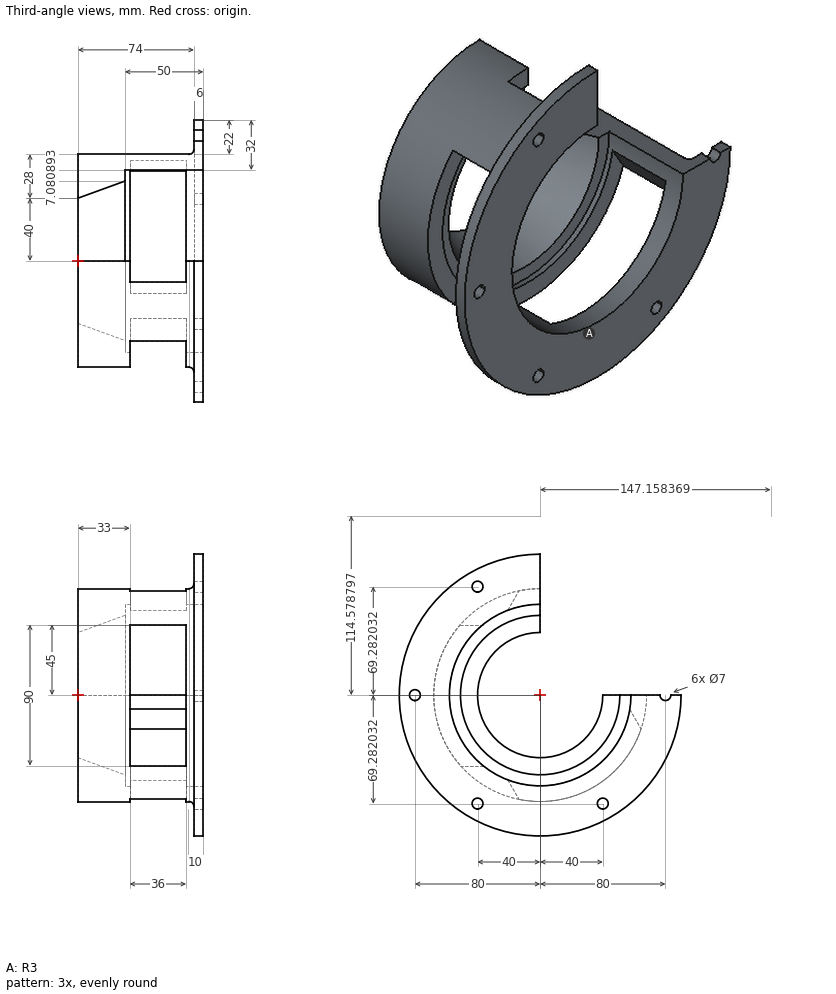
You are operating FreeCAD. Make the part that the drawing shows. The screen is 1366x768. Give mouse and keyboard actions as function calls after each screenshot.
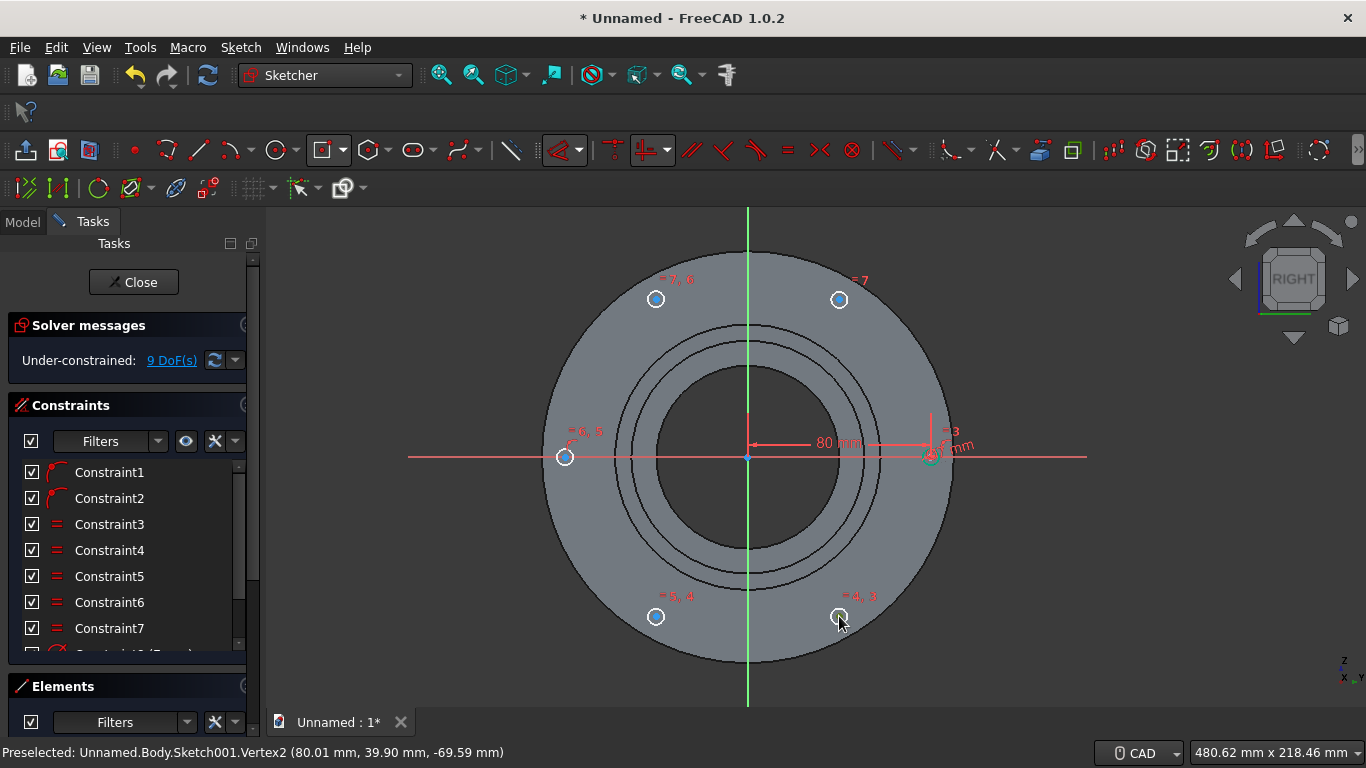
key(l)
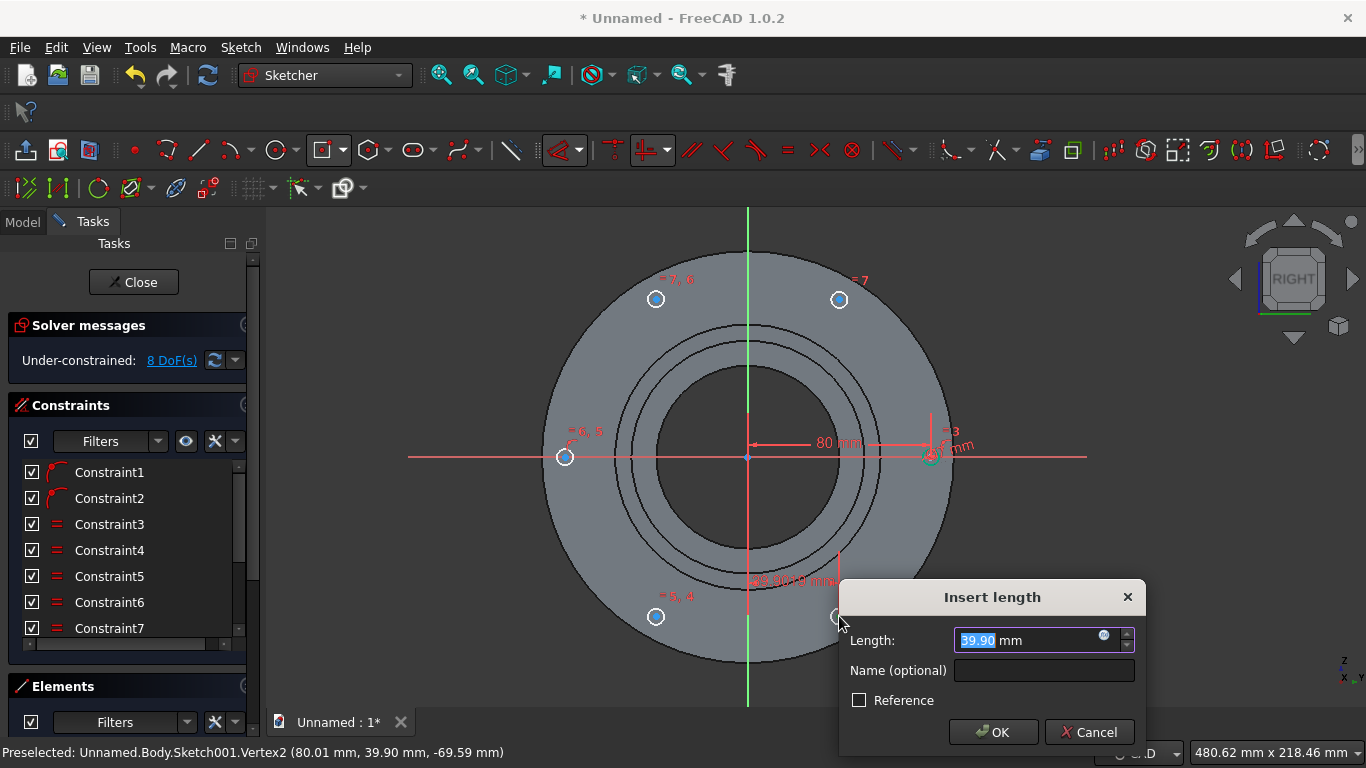
text(40)
key(Return)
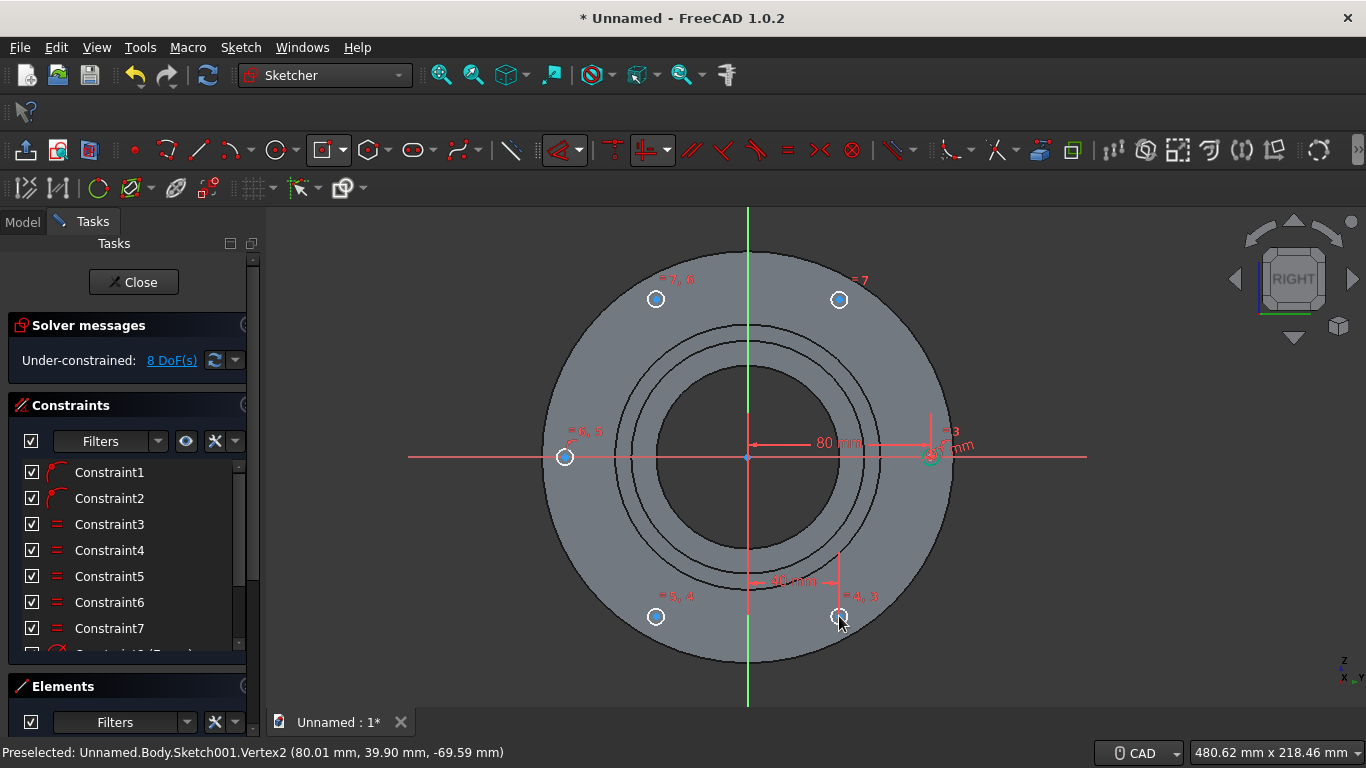
click(656, 617)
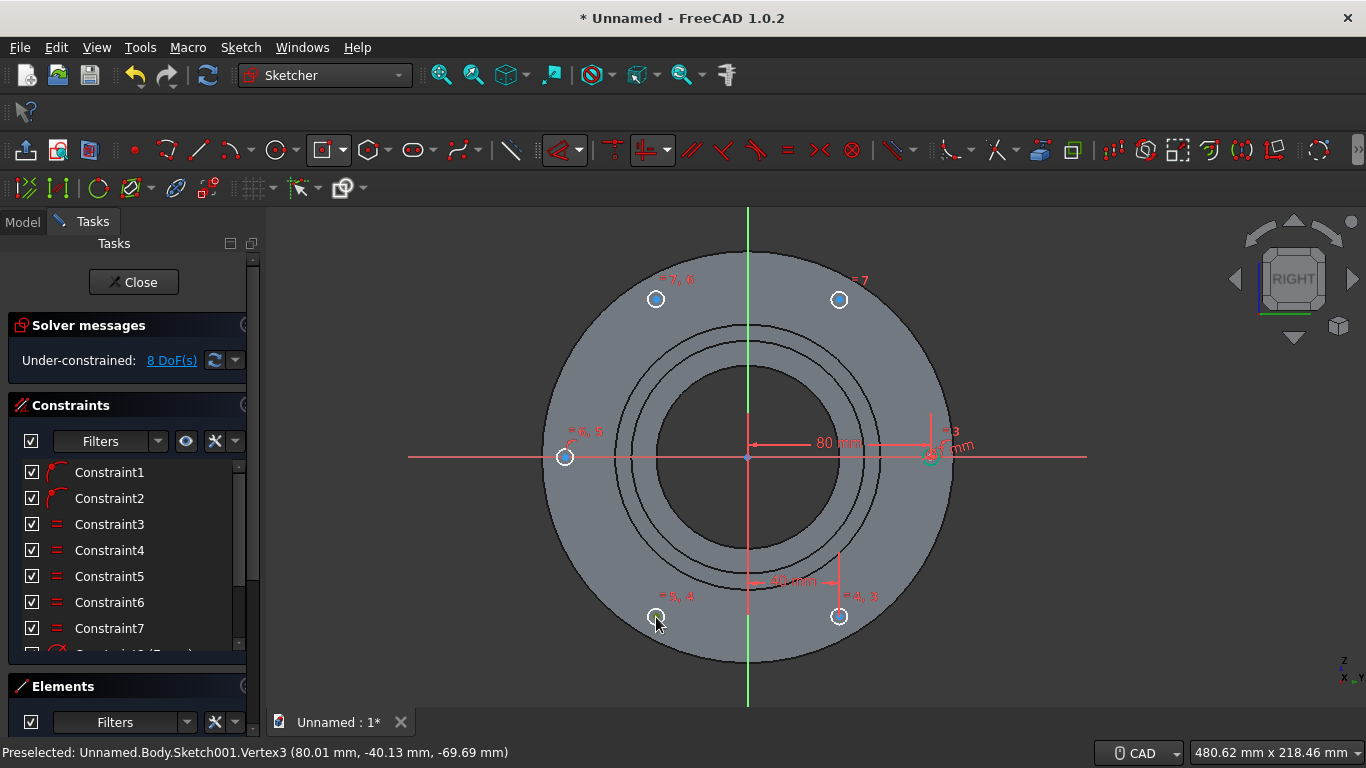
key(l)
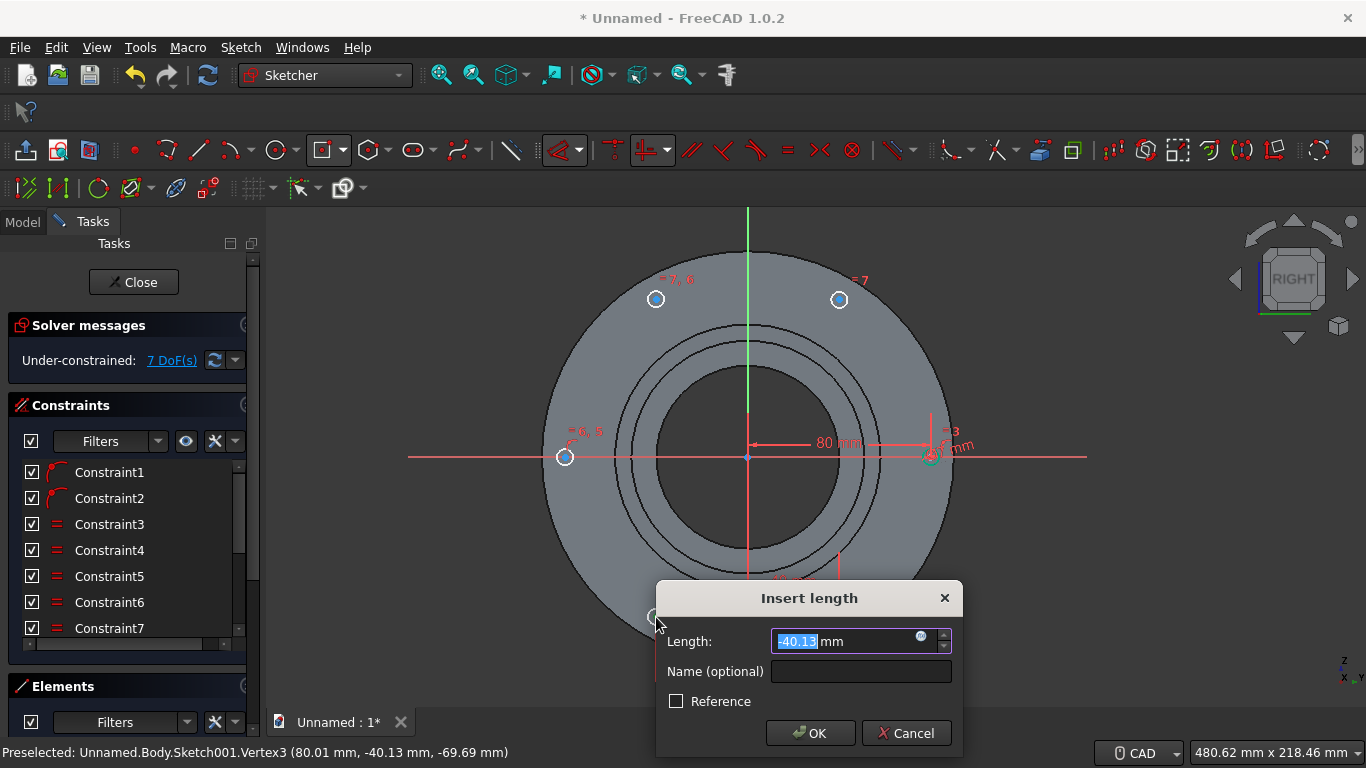
text(-40)
key(Return)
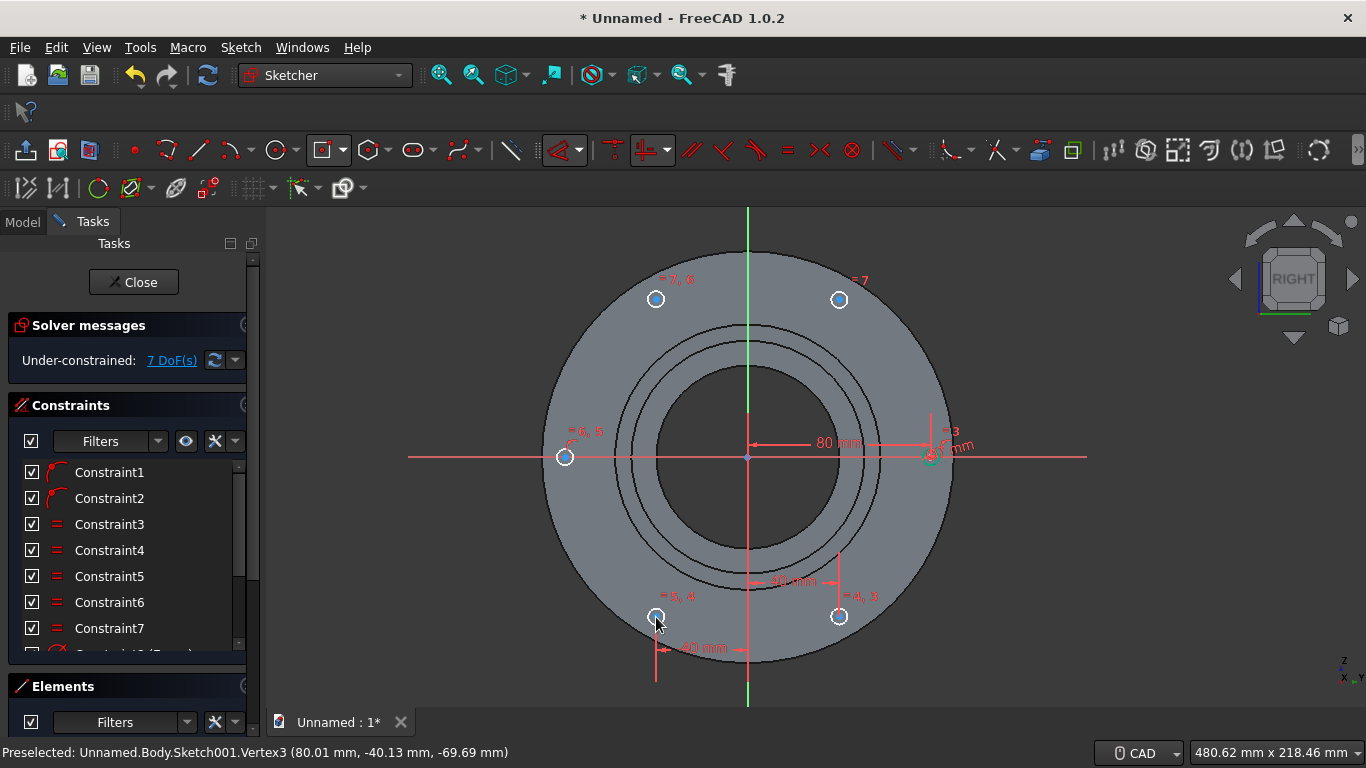
click(565, 457)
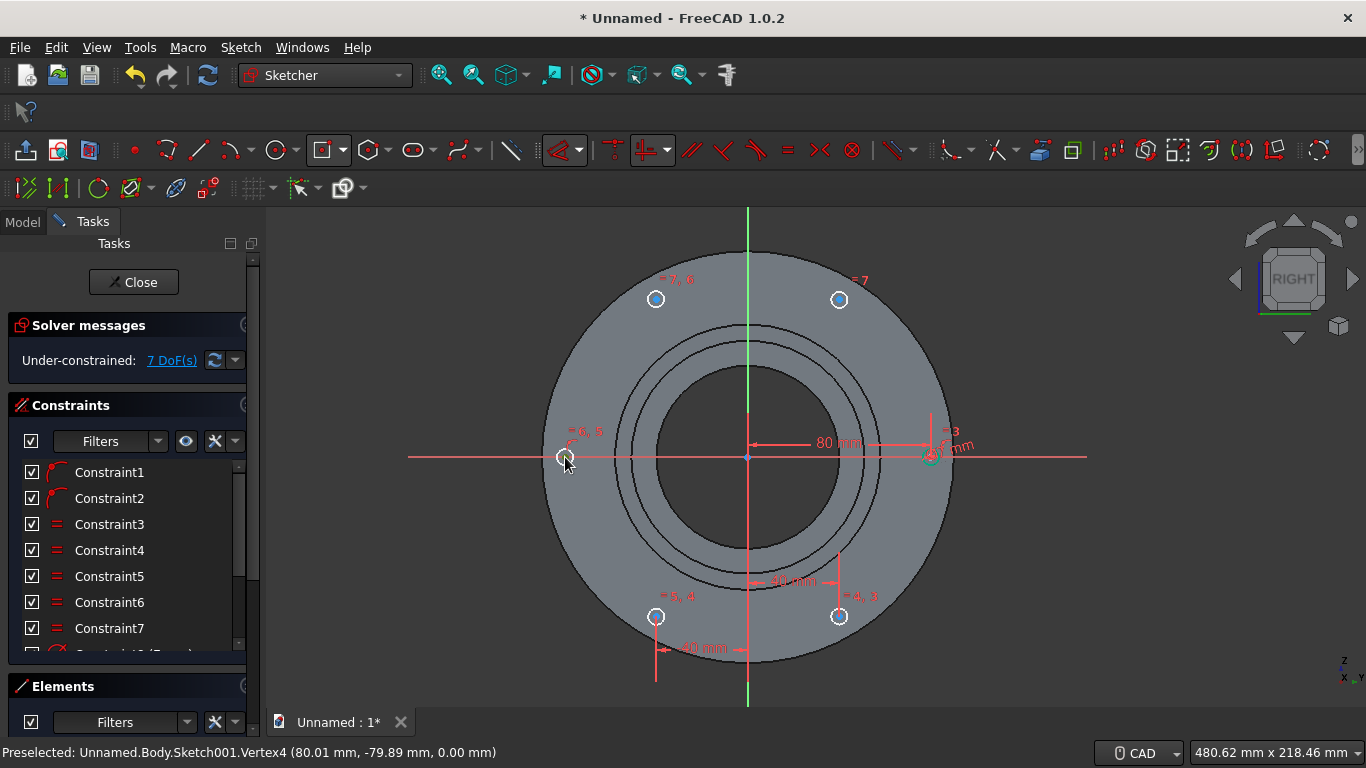
key(l)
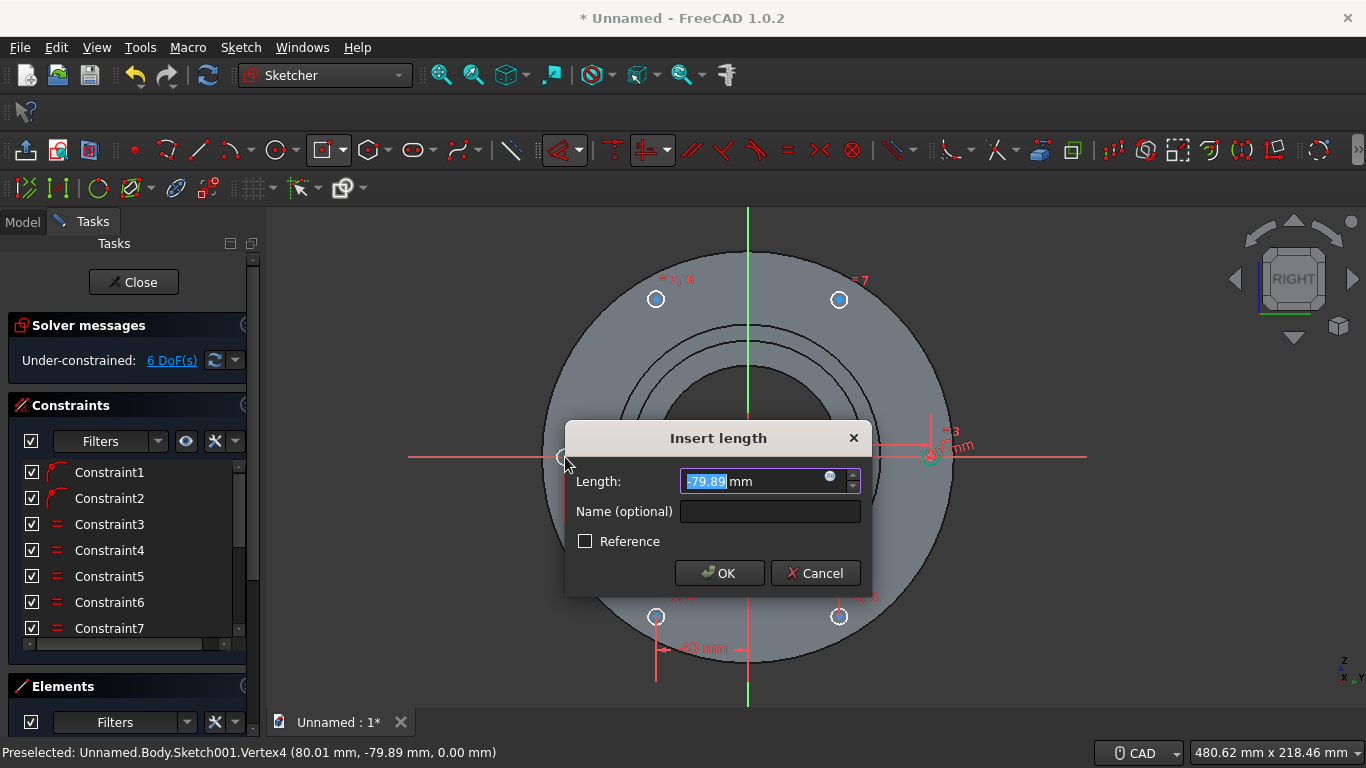
text(-80)
key(Return)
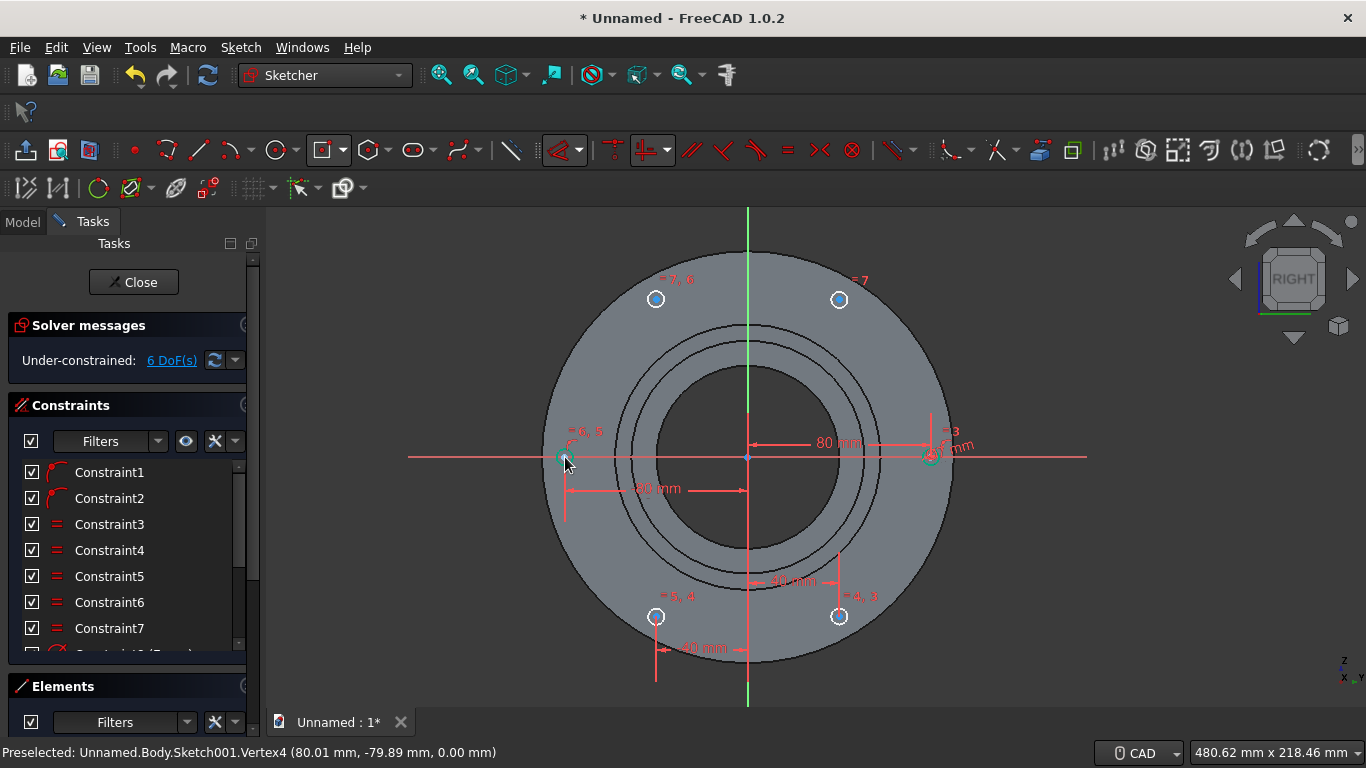
click(656, 299)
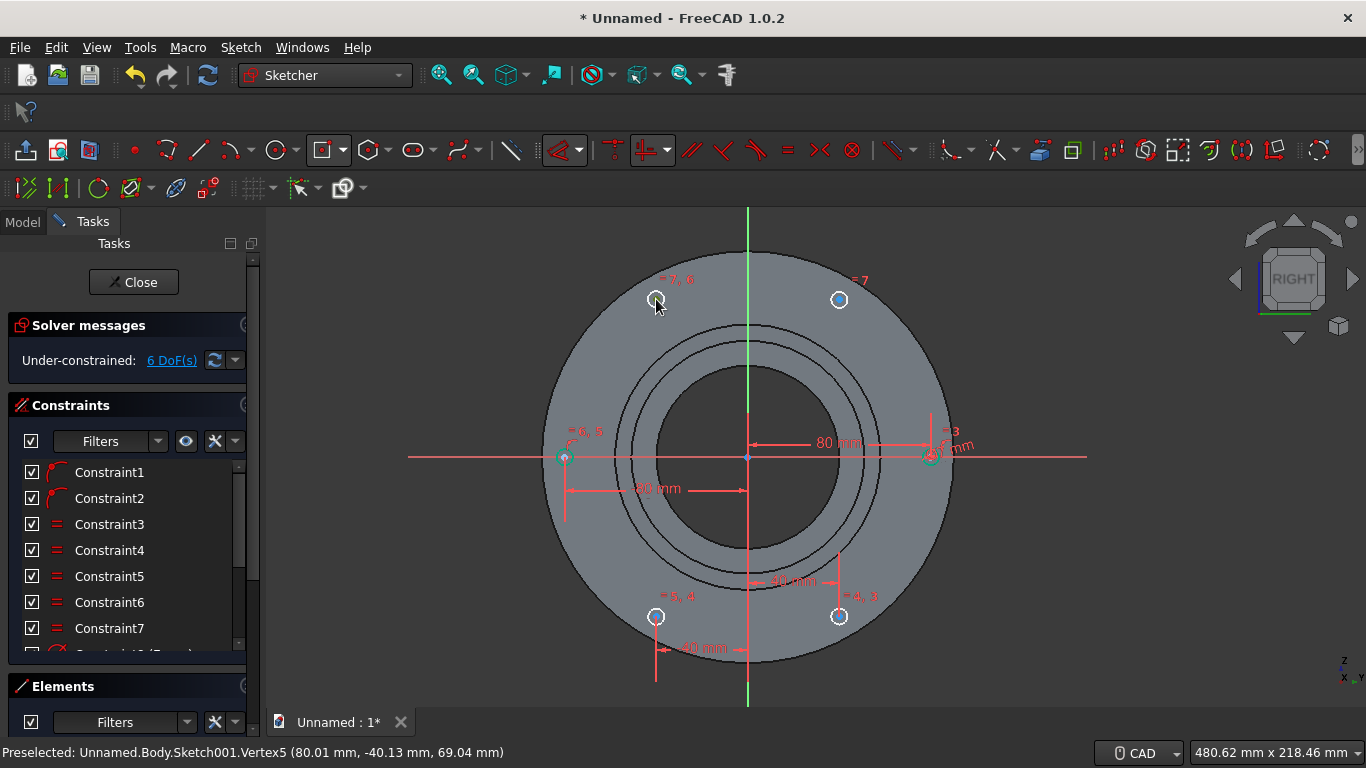
key(l)